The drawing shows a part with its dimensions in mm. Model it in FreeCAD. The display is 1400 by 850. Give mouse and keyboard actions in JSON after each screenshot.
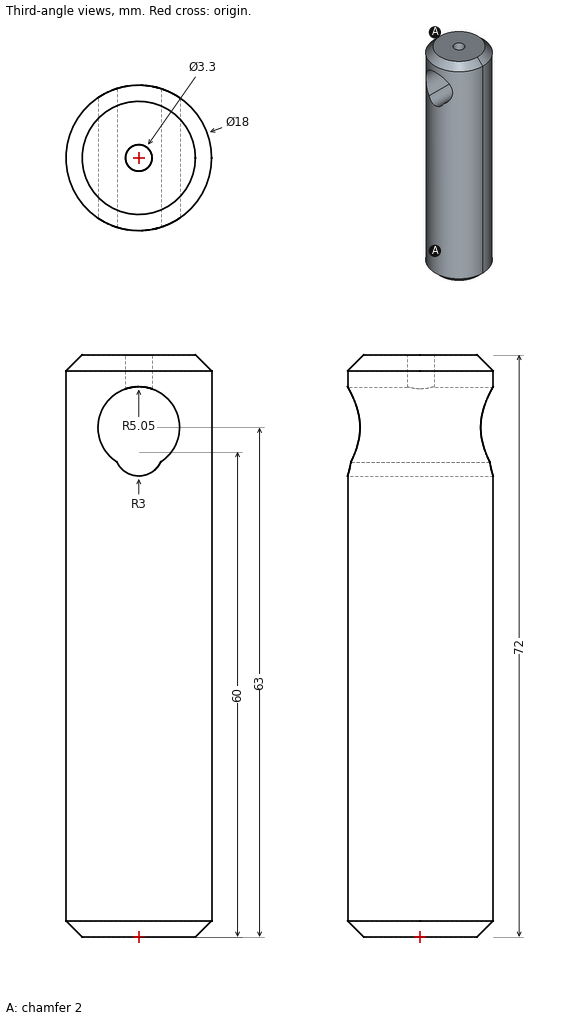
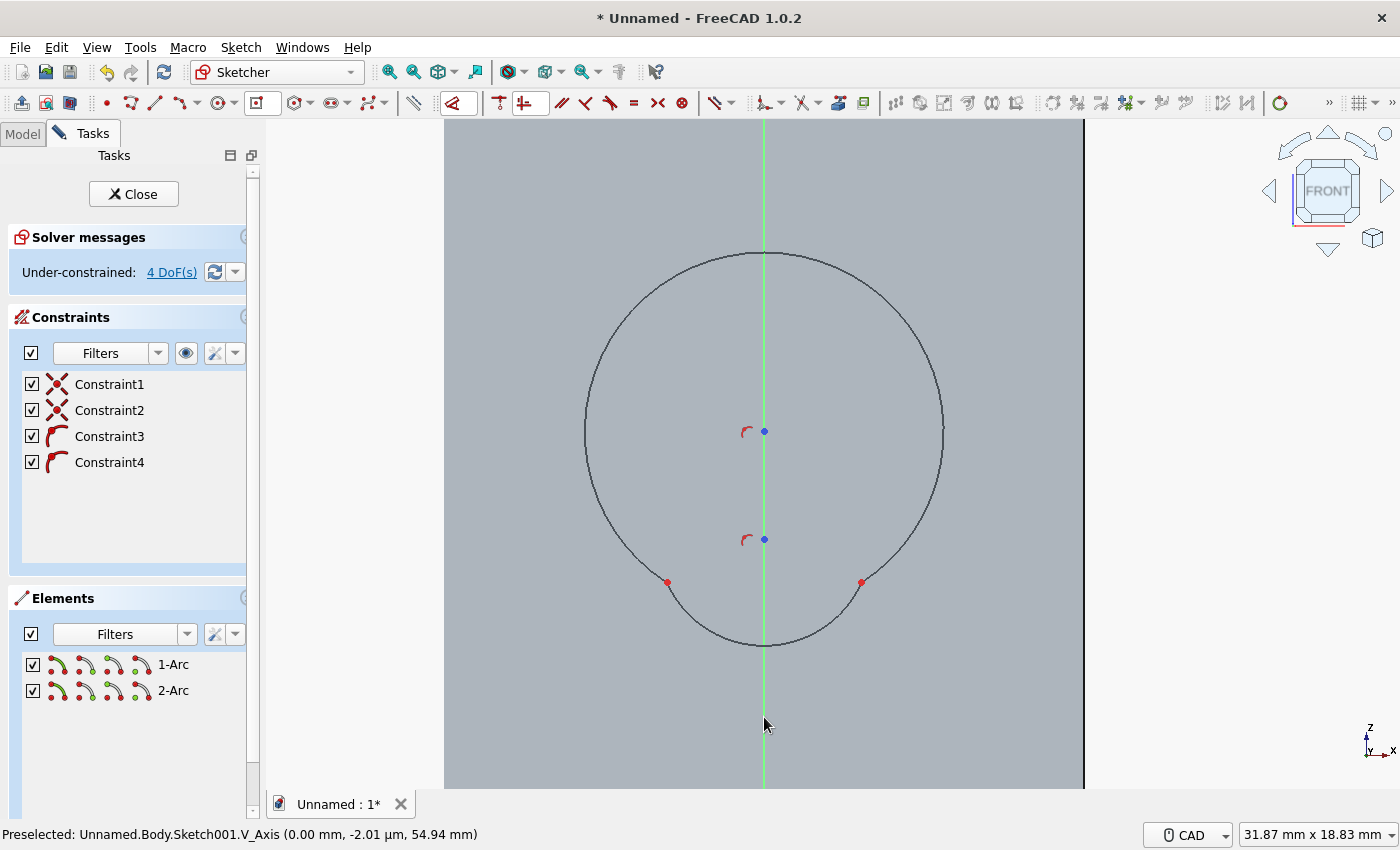
{"action": "left_click", "coordinate": [918, 339]}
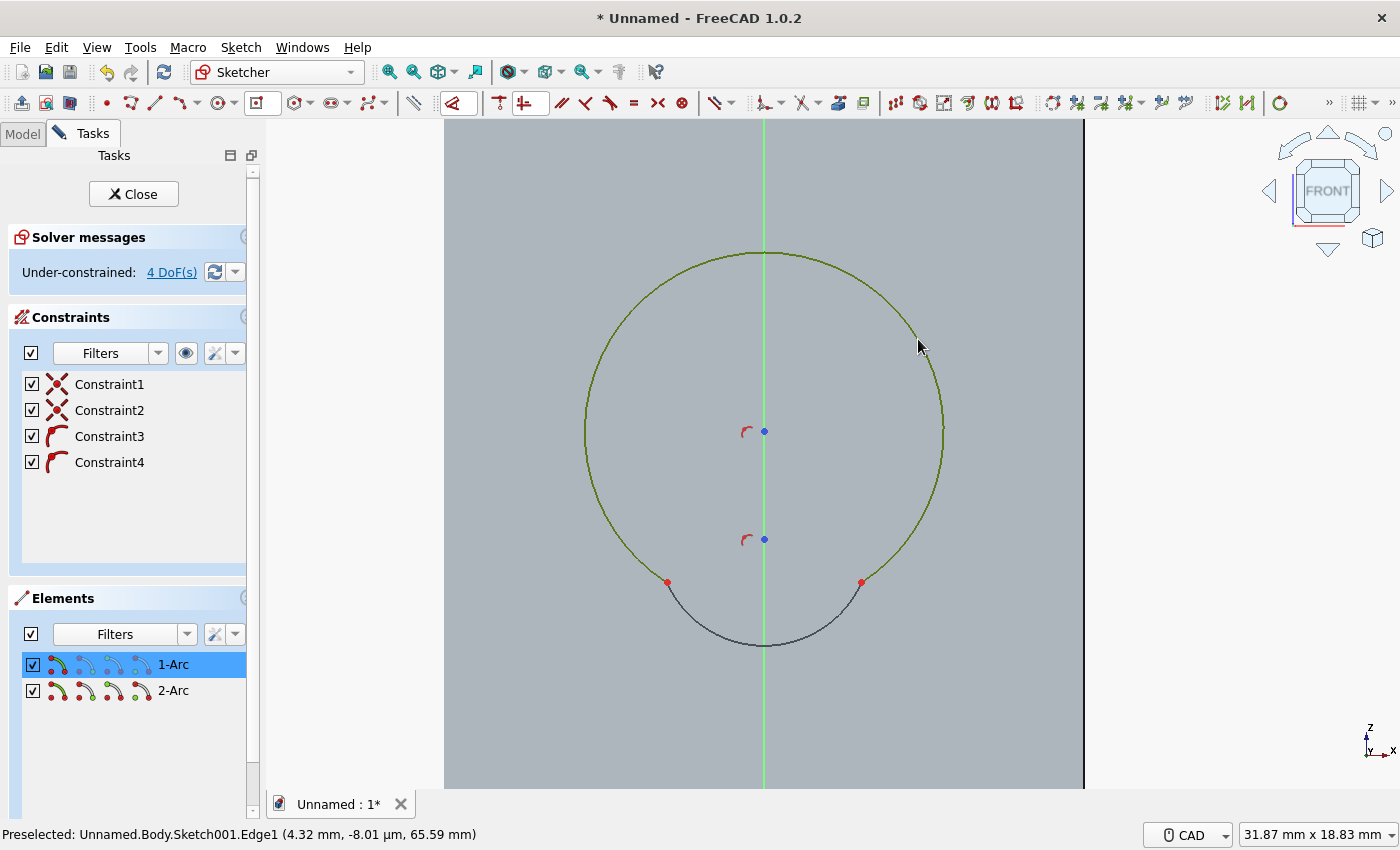
{"action": "left_click", "coordinate": [472, 104]}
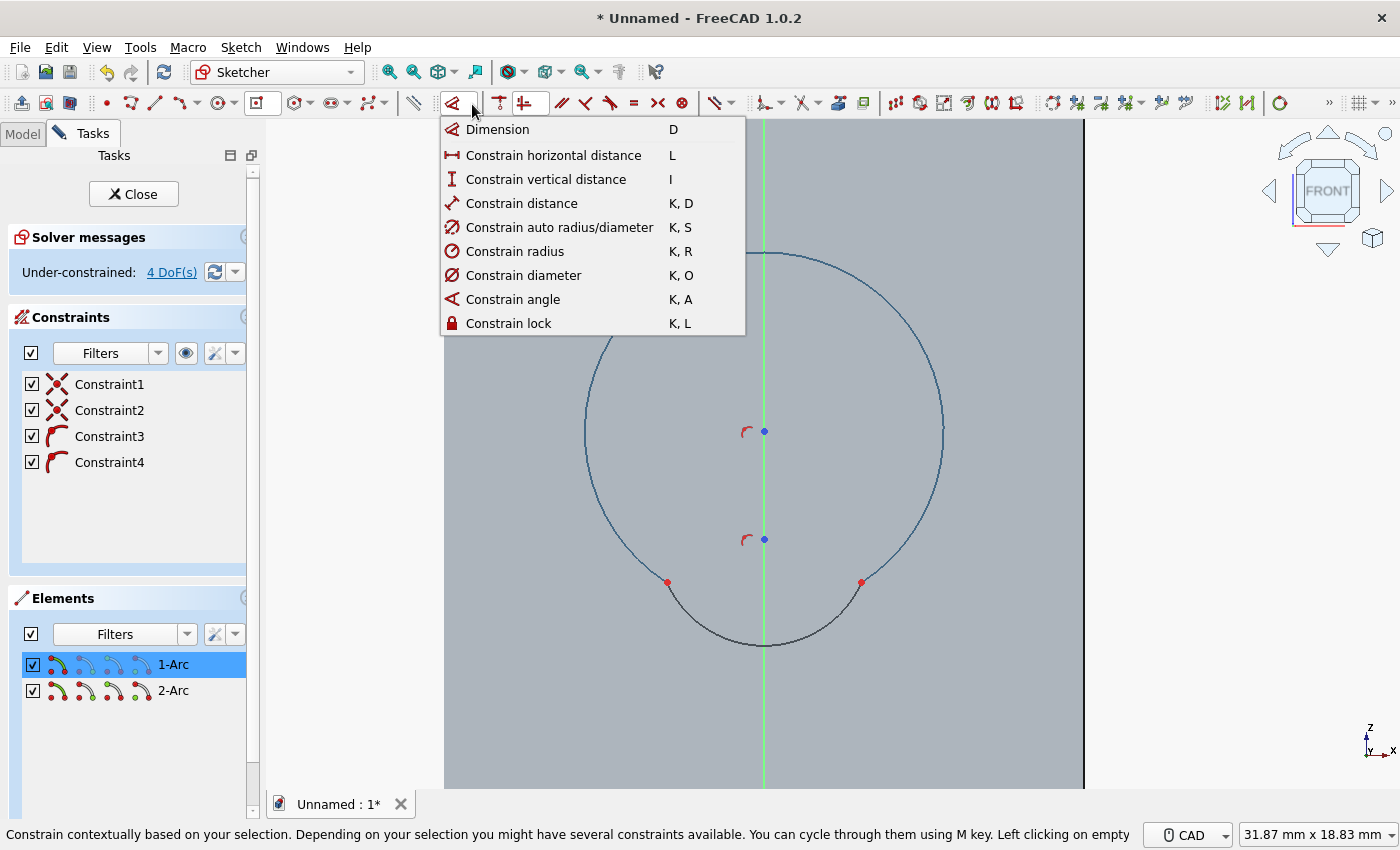
{"action": "left_click", "coordinate": [593, 251]}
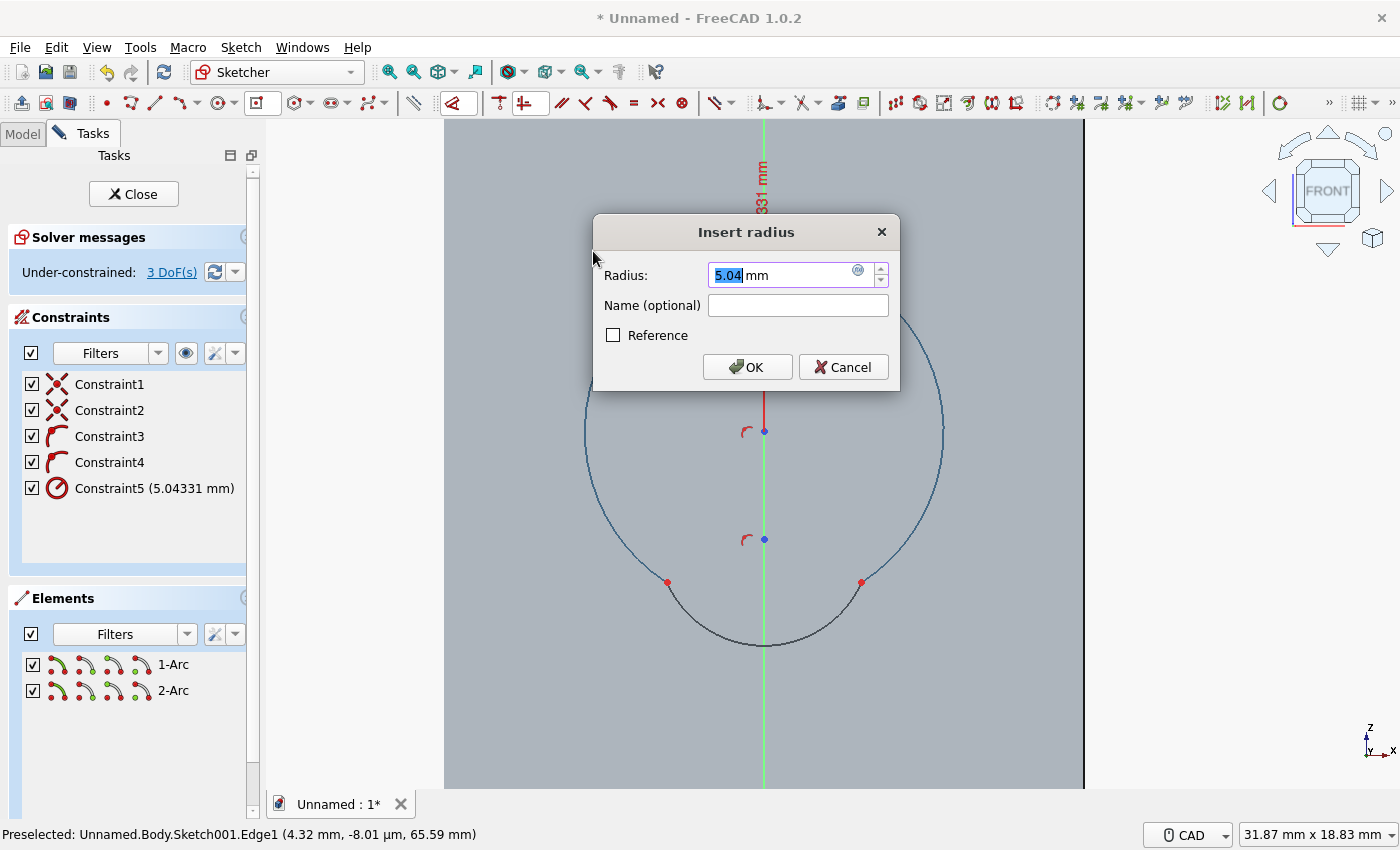
{"action": "type", "text": "5.05"}
{"action": "key", "text": "Return"}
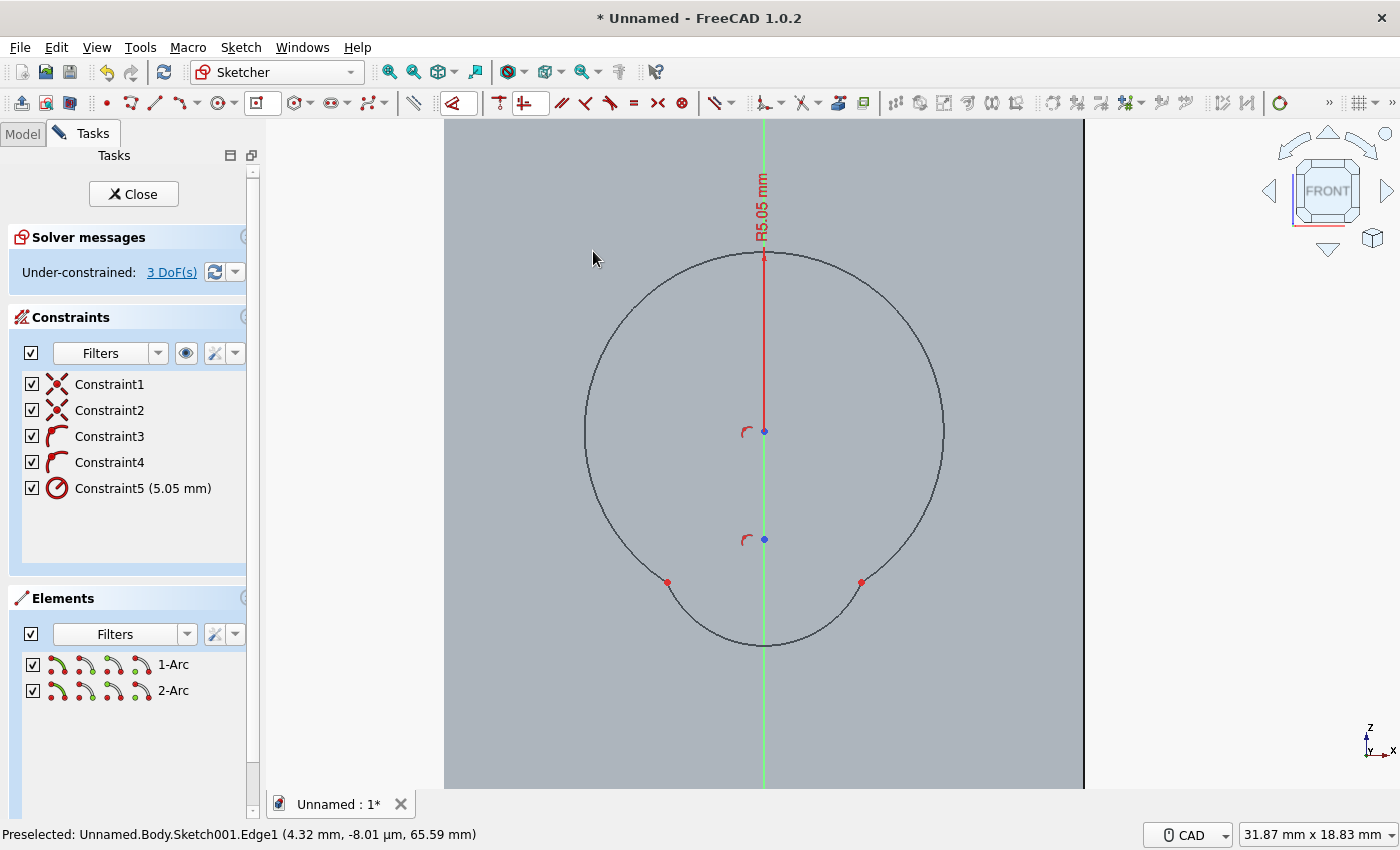
{"action": "left_click", "coordinate": [717, 635]}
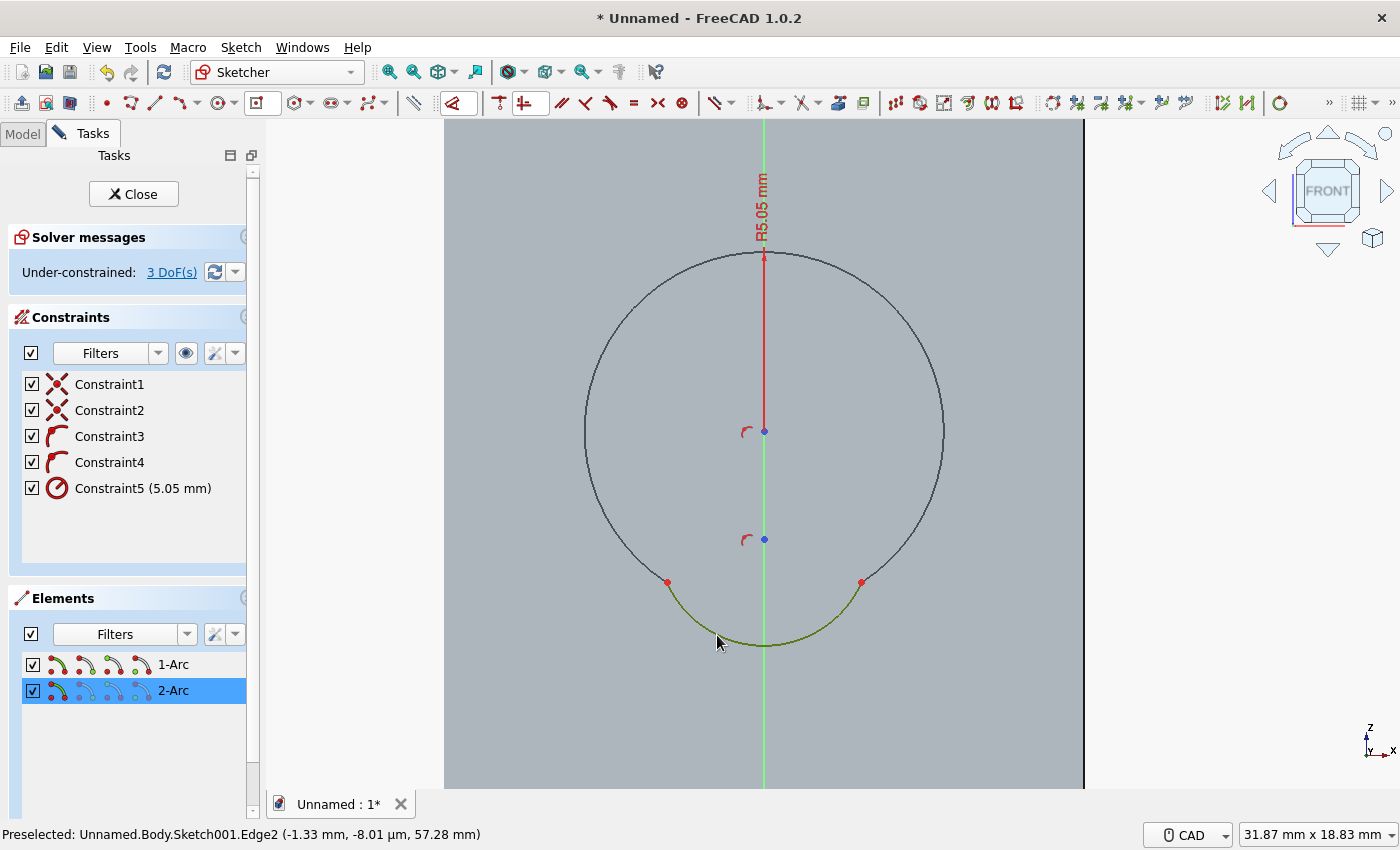
{"action": "key", "text": "k r"}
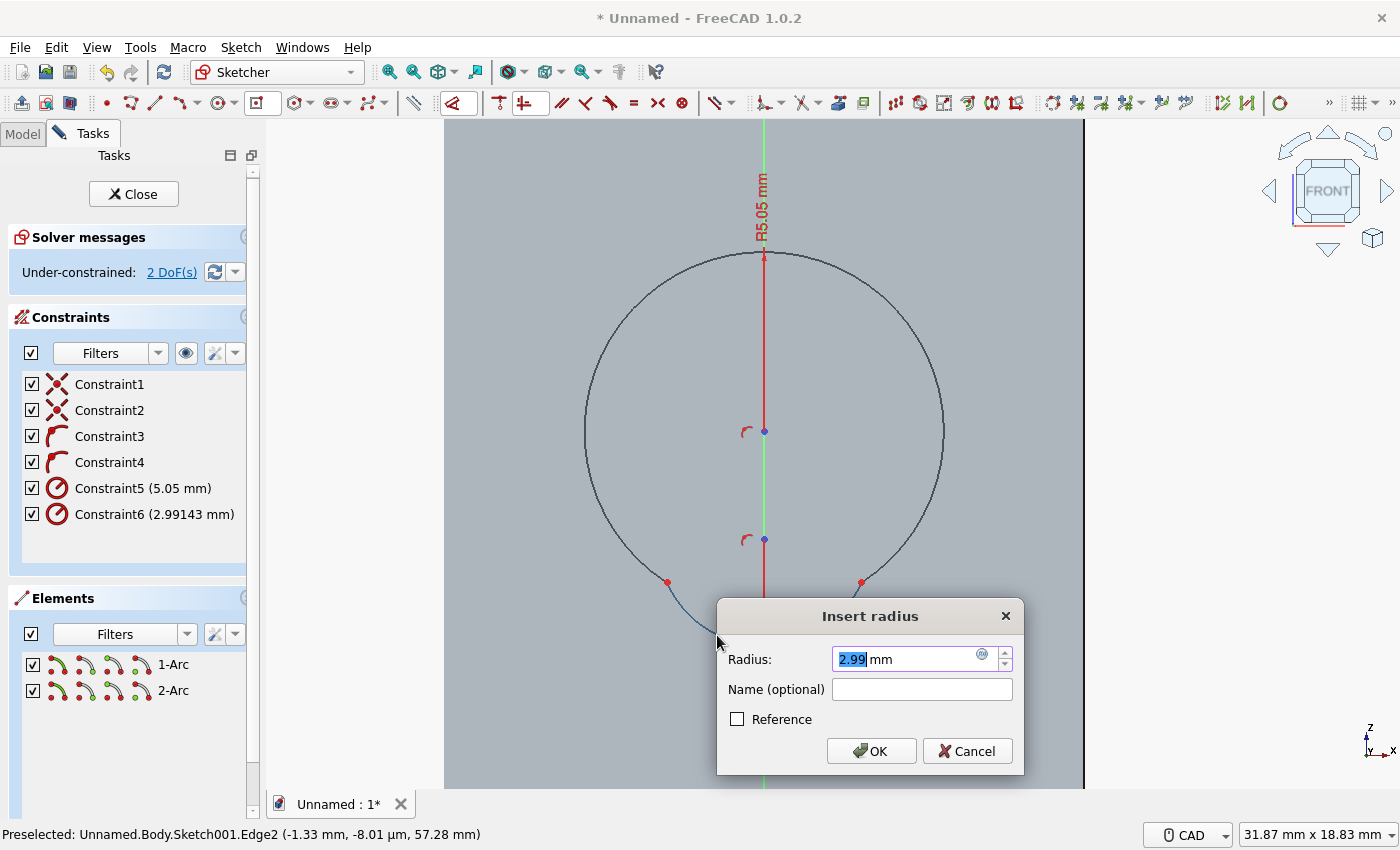
{"action": "type", "text": "3"}
{"action": "key", "text": "Return"}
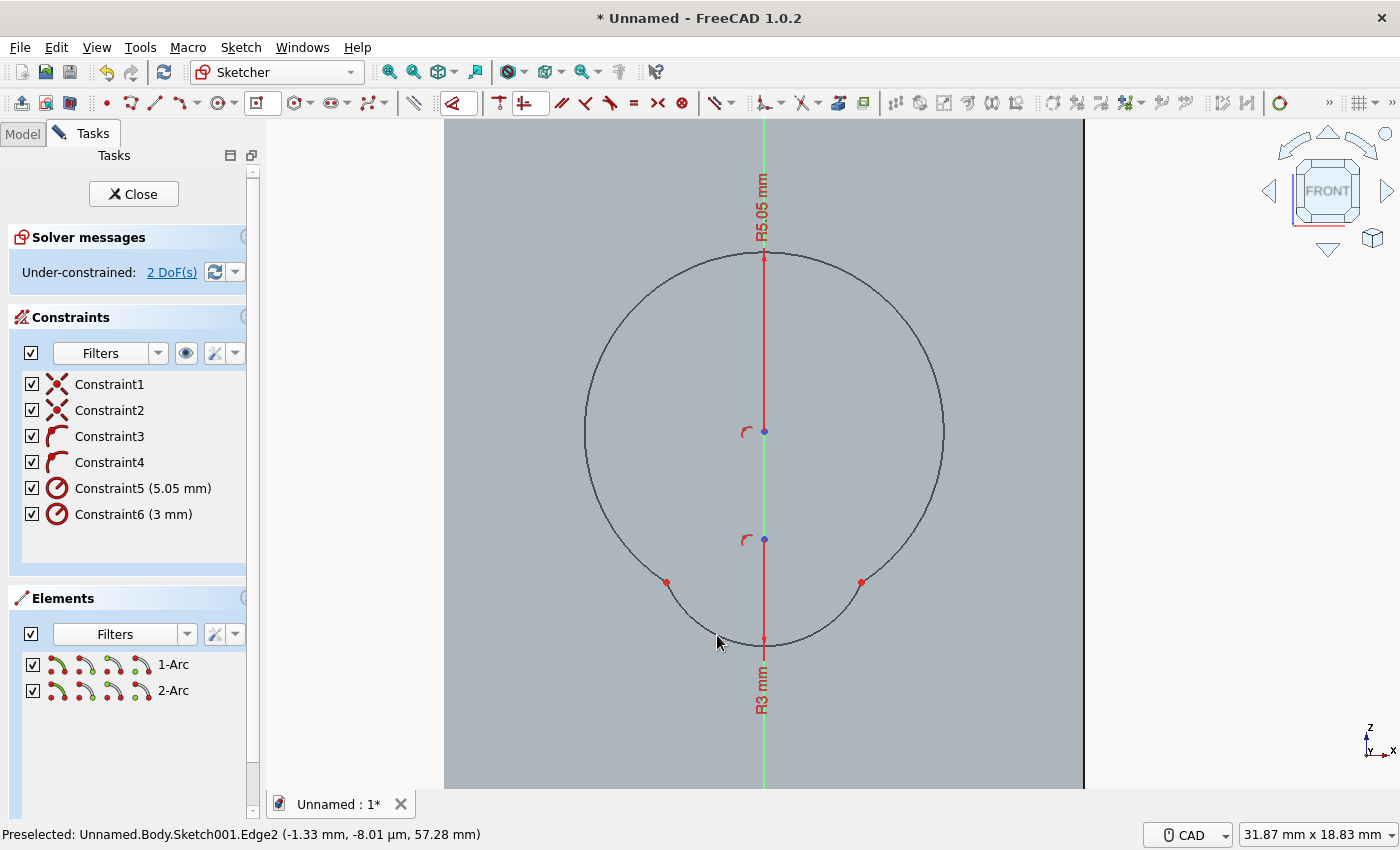
{"action": "left_click", "coordinate": [764, 432]}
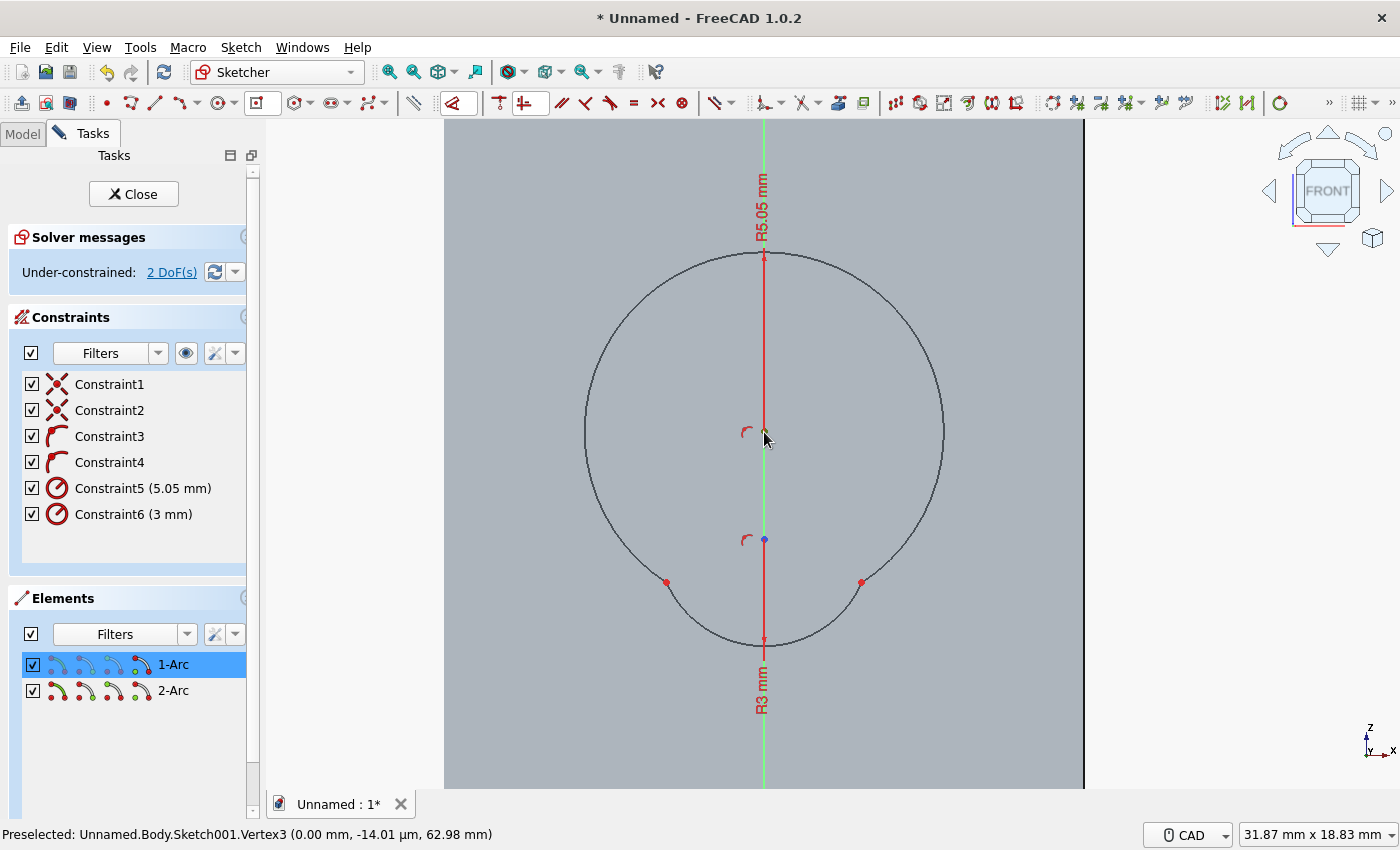
{"action": "key", "text": "i"}